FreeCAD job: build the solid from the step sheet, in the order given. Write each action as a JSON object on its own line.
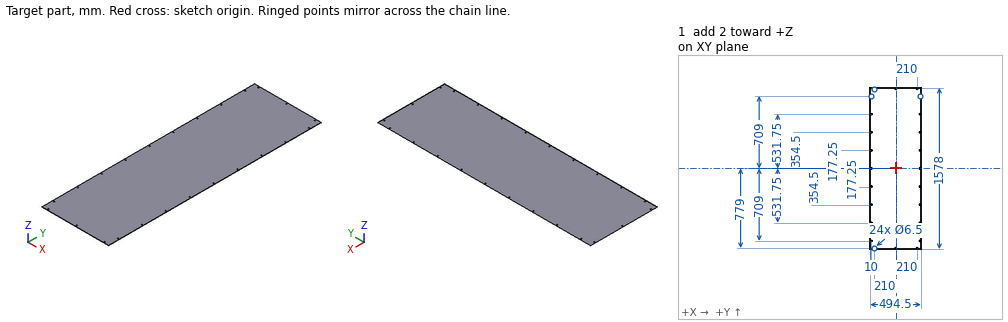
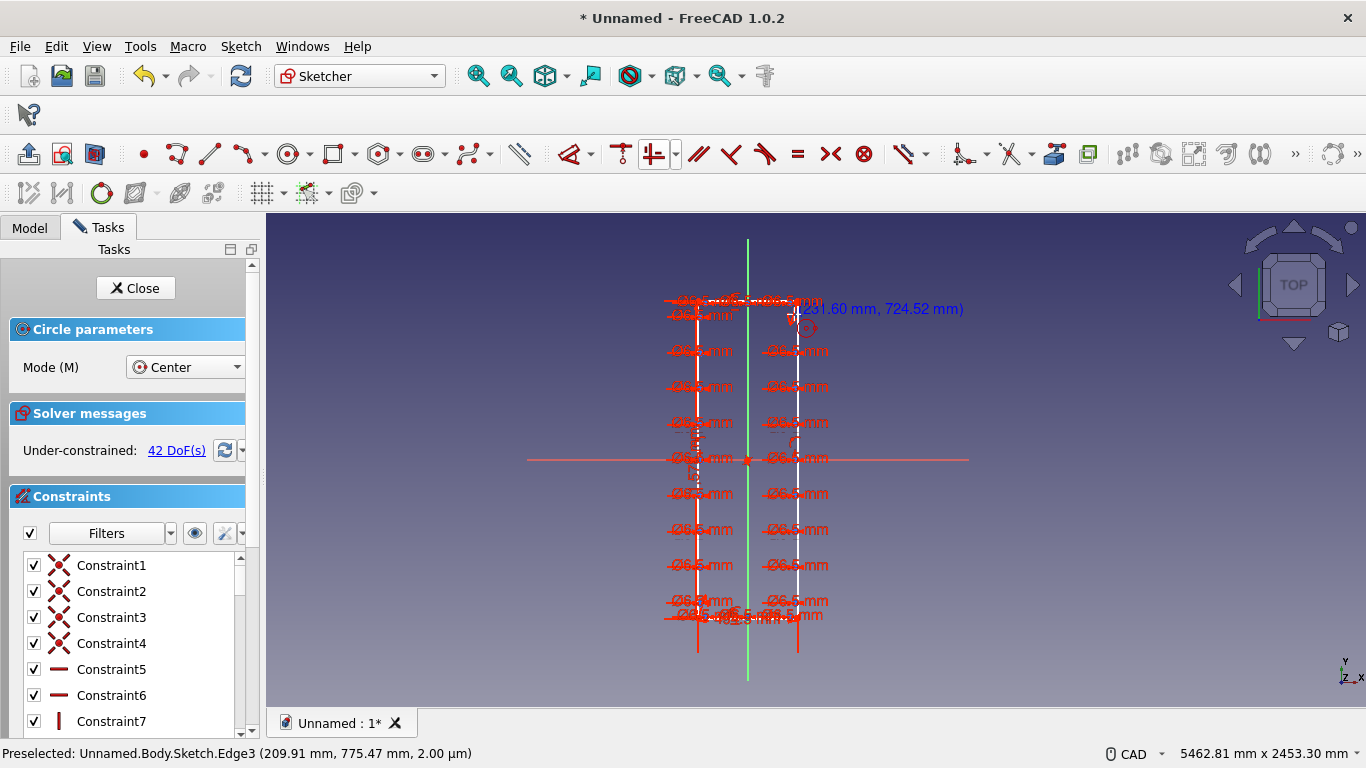
{"action": "scroll", "coordinate": [796, 317], "scroll_direction": "up", "scroll_amount": 11}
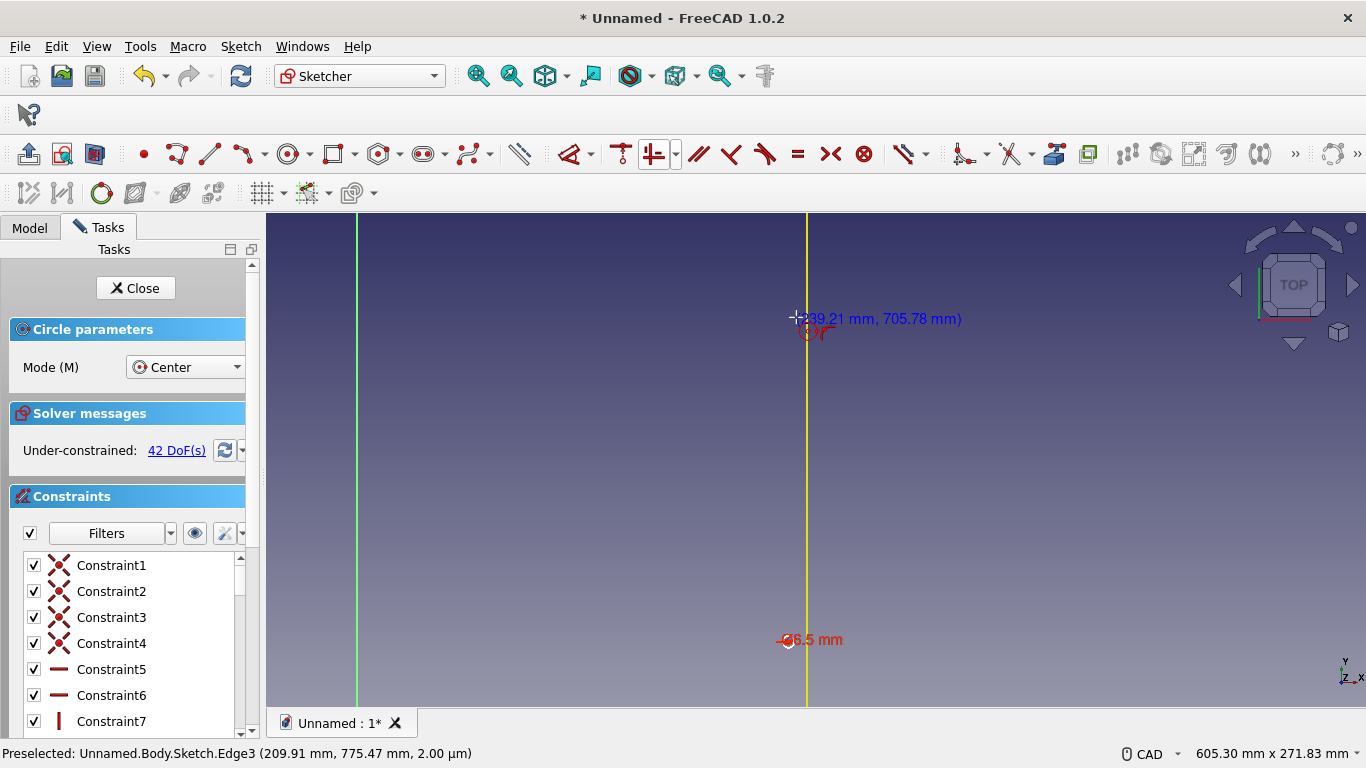
{"action": "left_click", "coordinate": [789, 318]}
{"action": "mouse_move", "coordinate": [784, 314]}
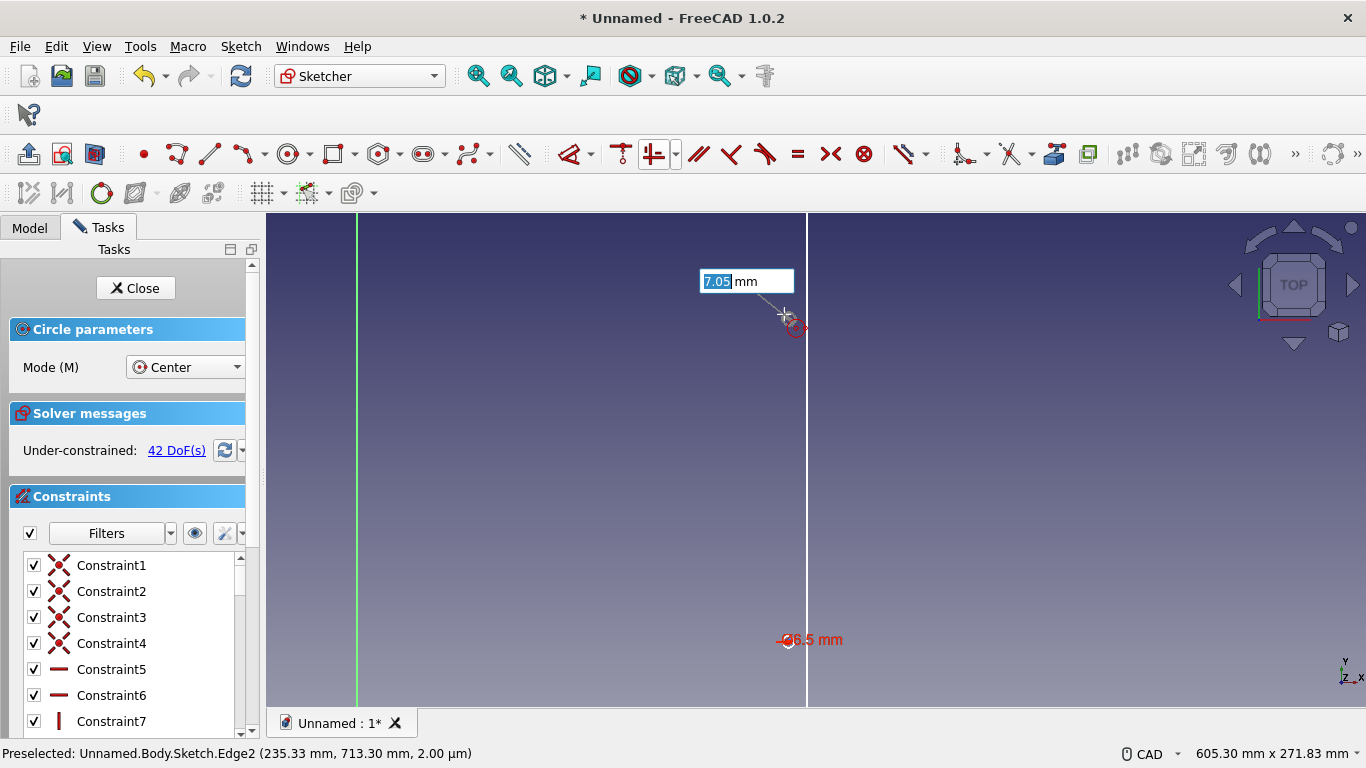
{"action": "type", "text": "6.5"}
{"action": "key", "text": "Return"}
{"action": "key", "text": "Escape"}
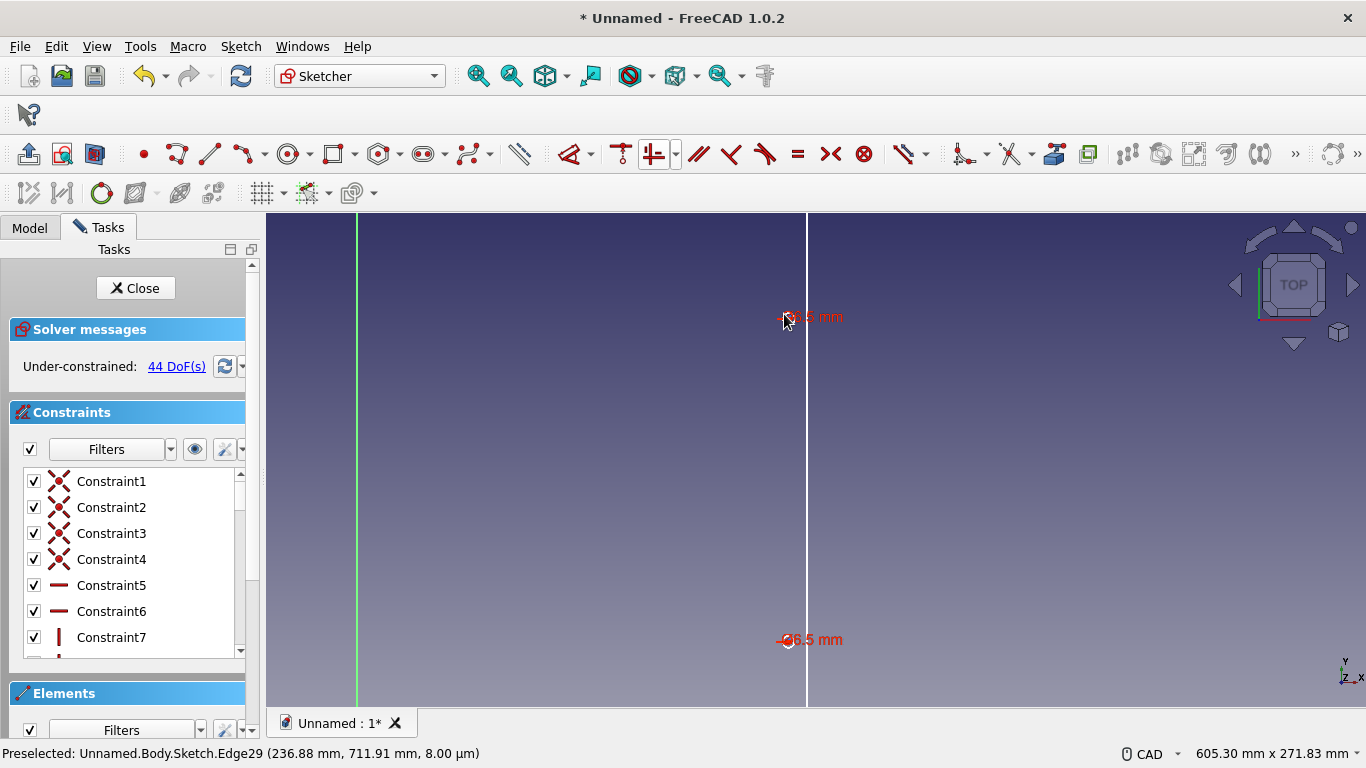
{"action": "scroll", "coordinate": [796, 317], "scroll_direction": "down", "scroll_amount": 11}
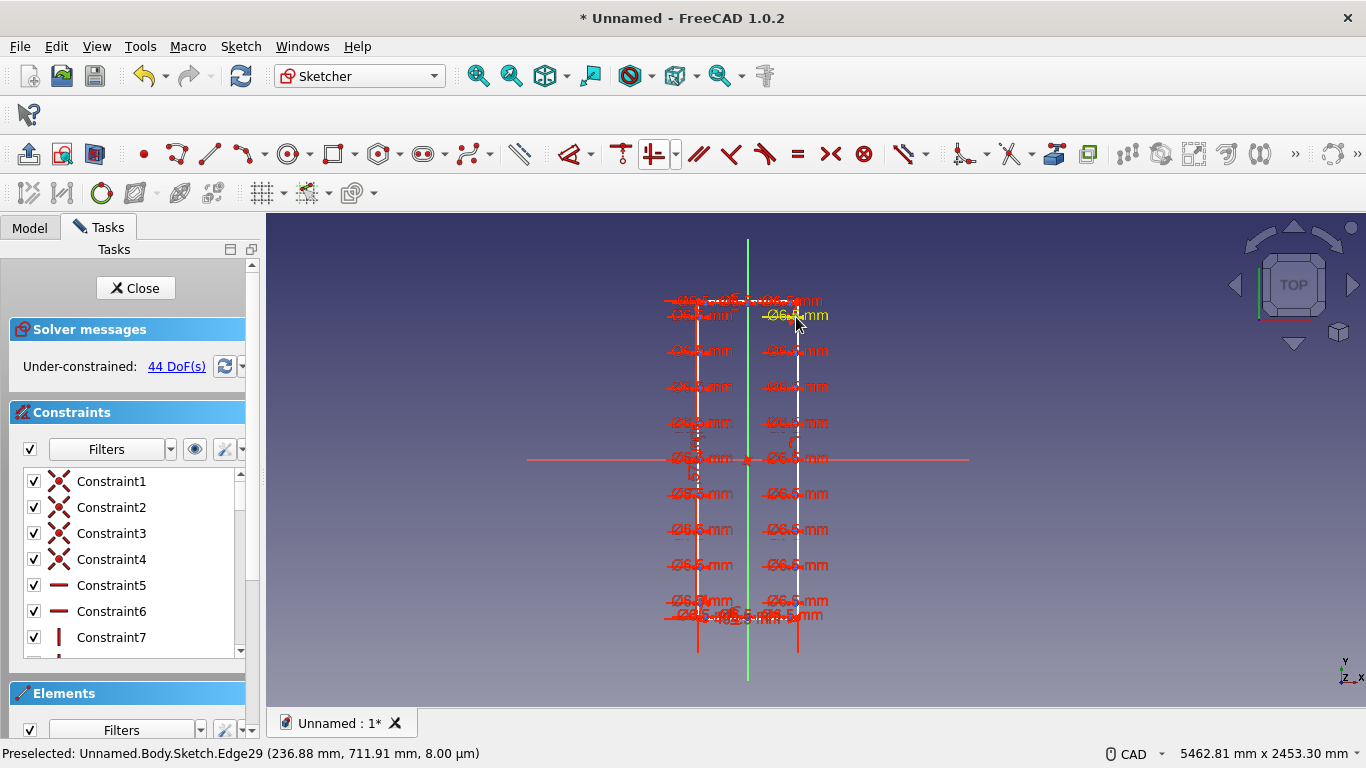
{"action": "left_click", "coordinate": [700, 603]}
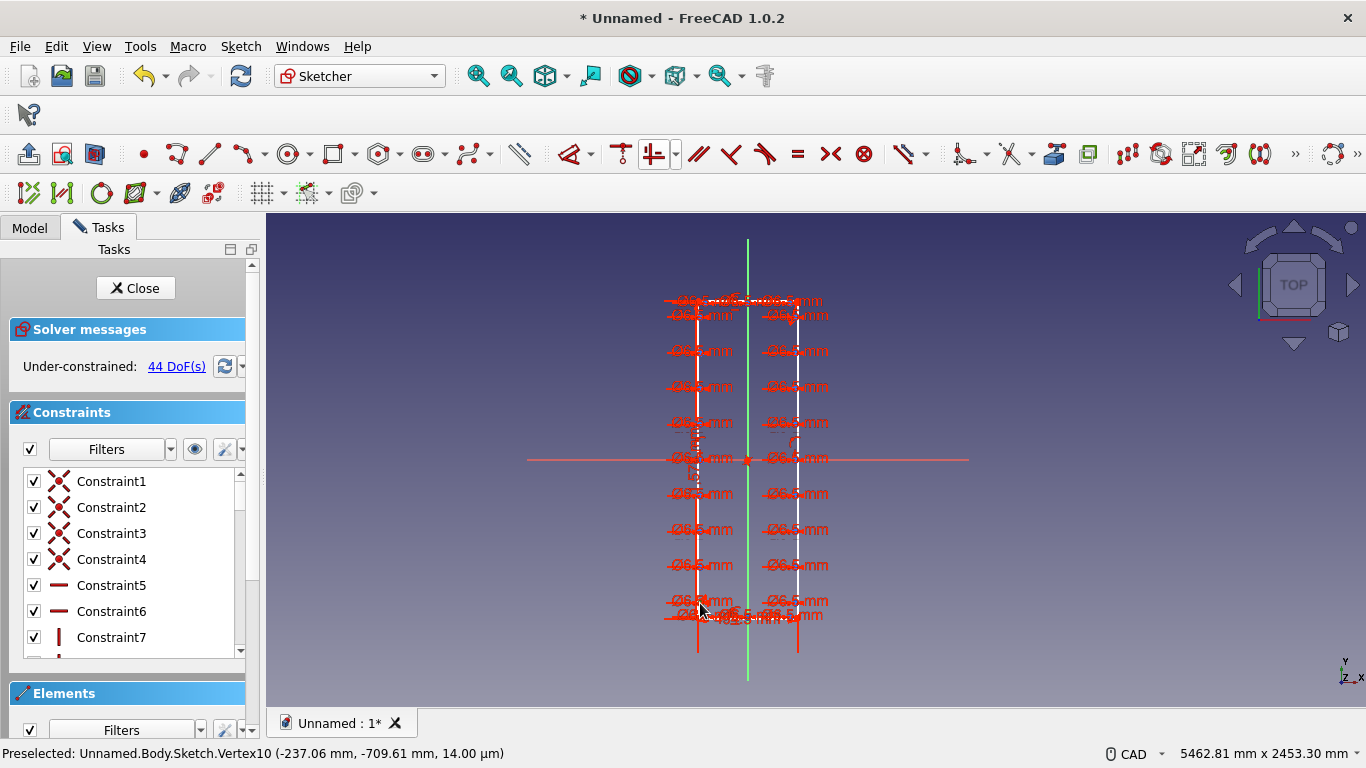
{"action": "left_click", "coordinate": [700, 567]}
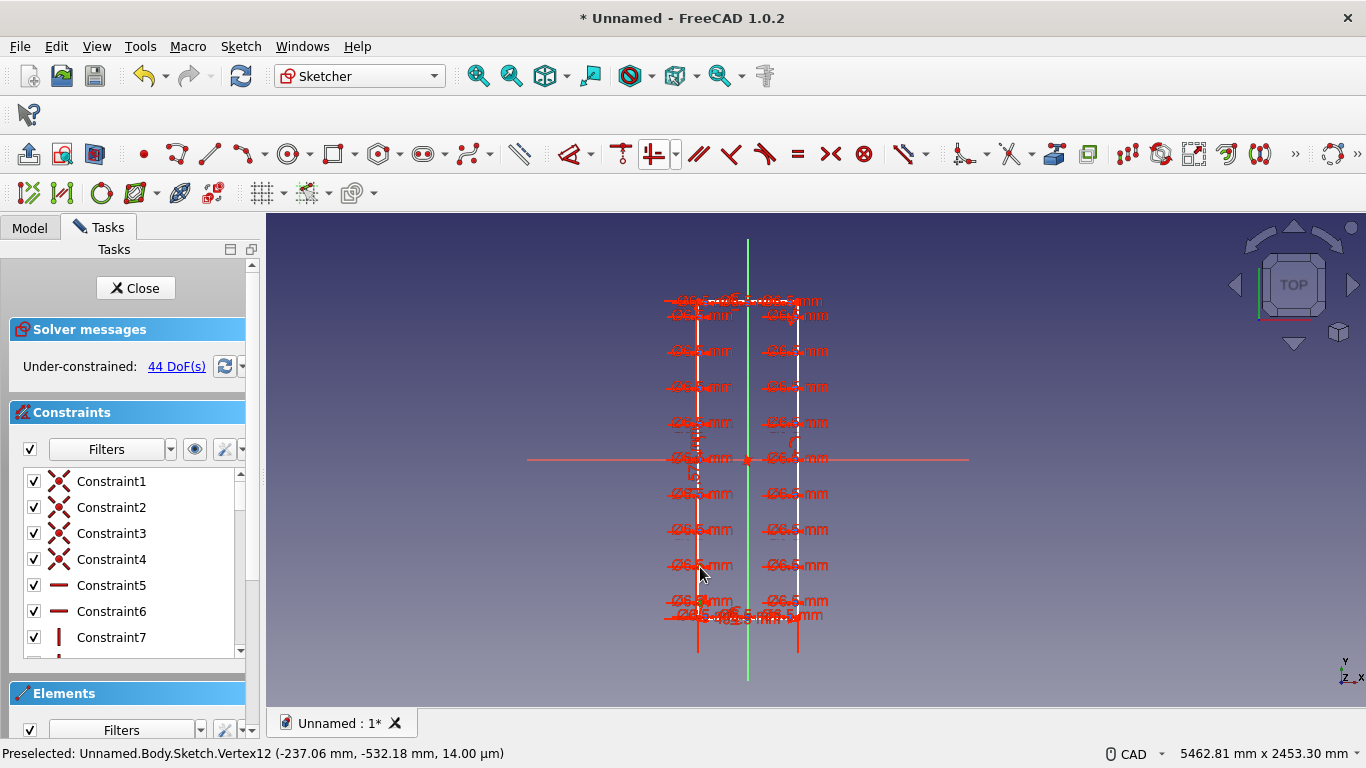
{"action": "key", "text": "v"}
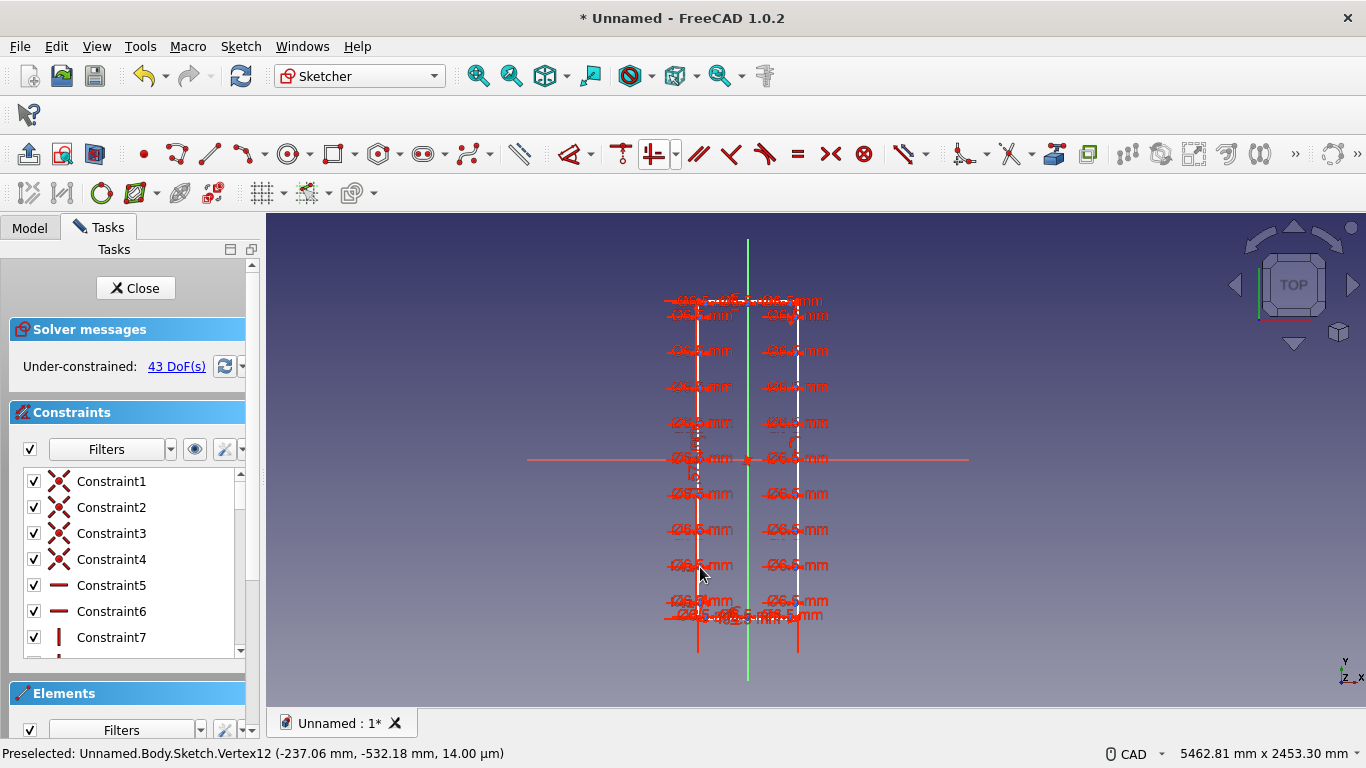
{"action": "left_click", "coordinate": [700, 567]}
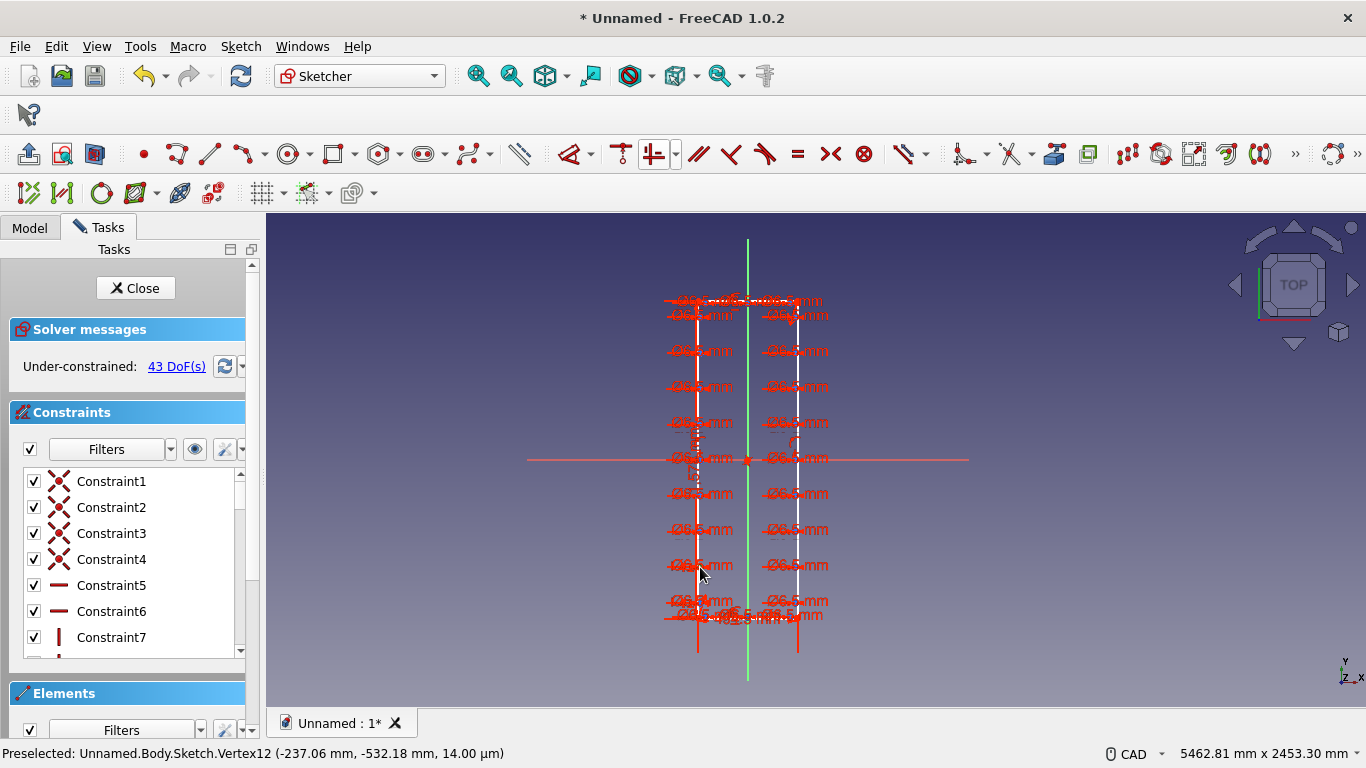
{"action": "left_click", "coordinate": [700, 532]}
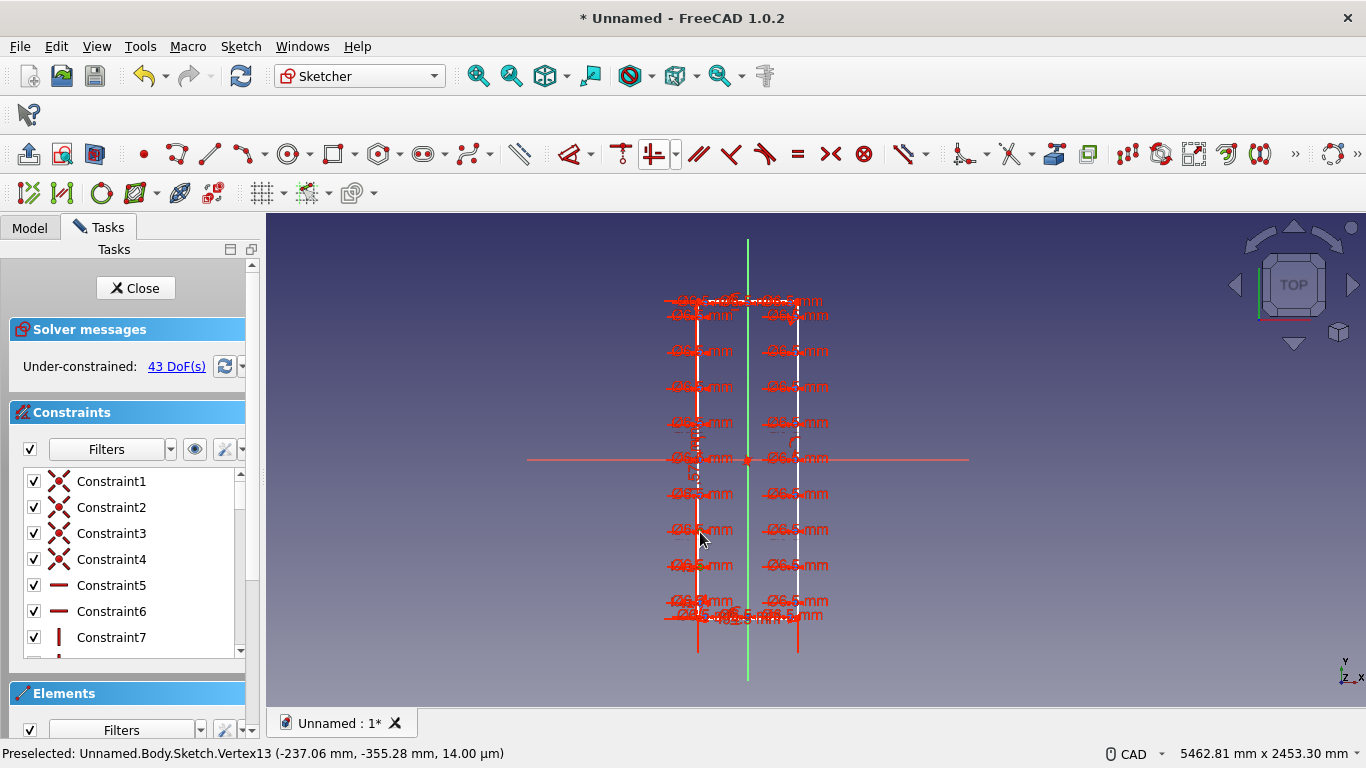
{"action": "key", "text": "v"}